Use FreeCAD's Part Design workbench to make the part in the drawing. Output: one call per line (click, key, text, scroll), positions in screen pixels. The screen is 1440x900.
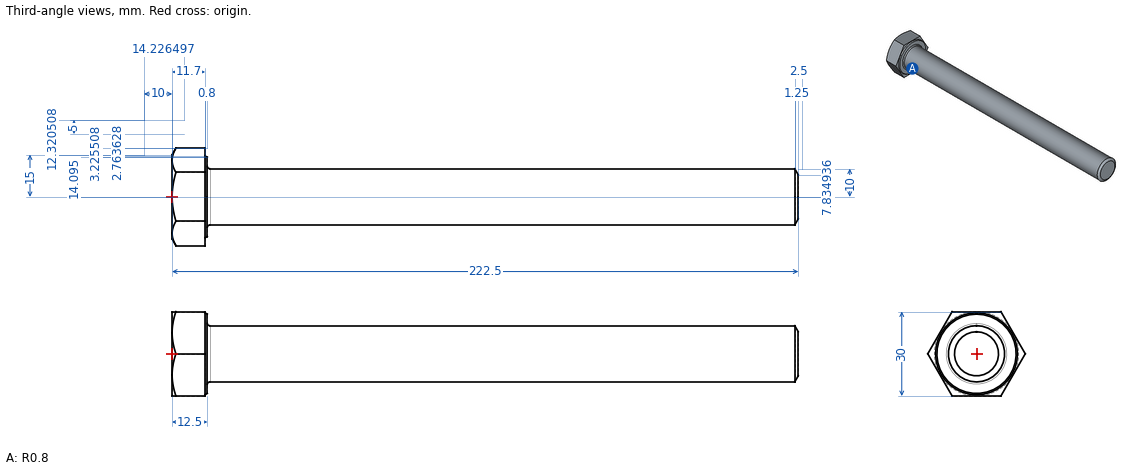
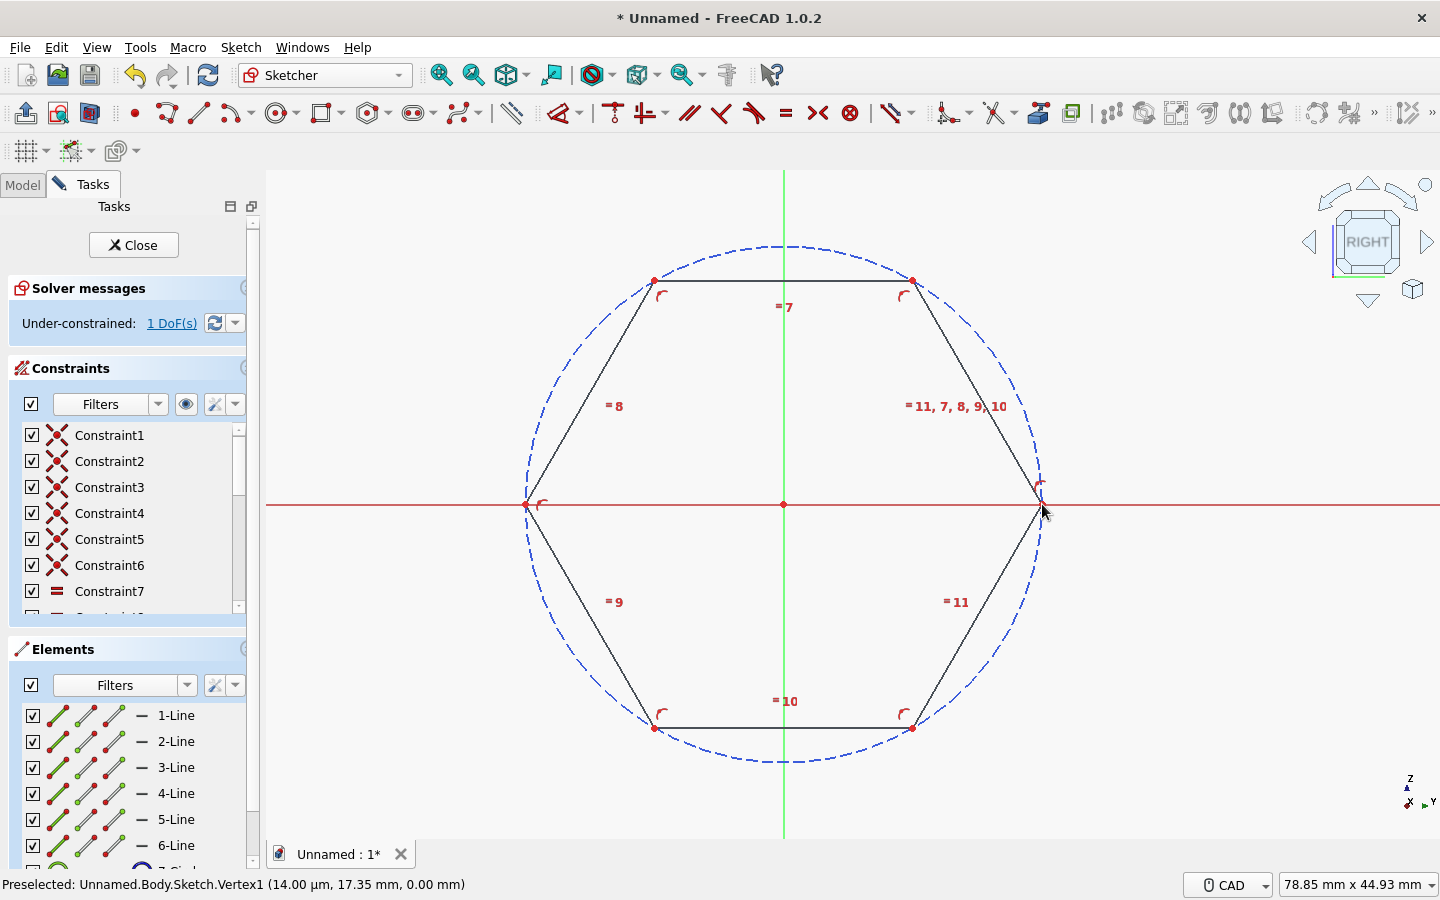
click(558, 114)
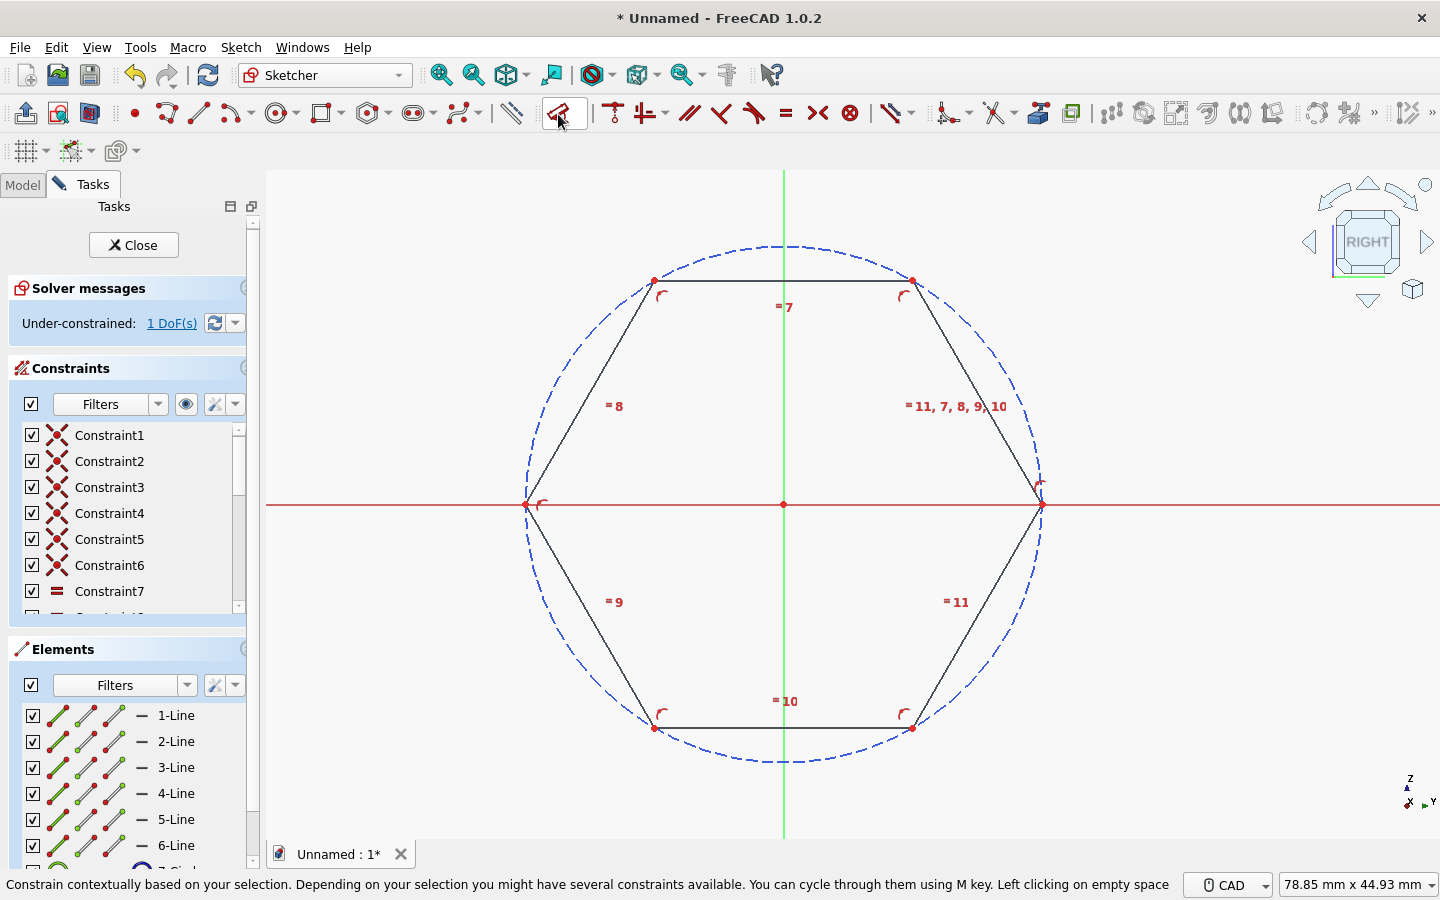
click(655, 728)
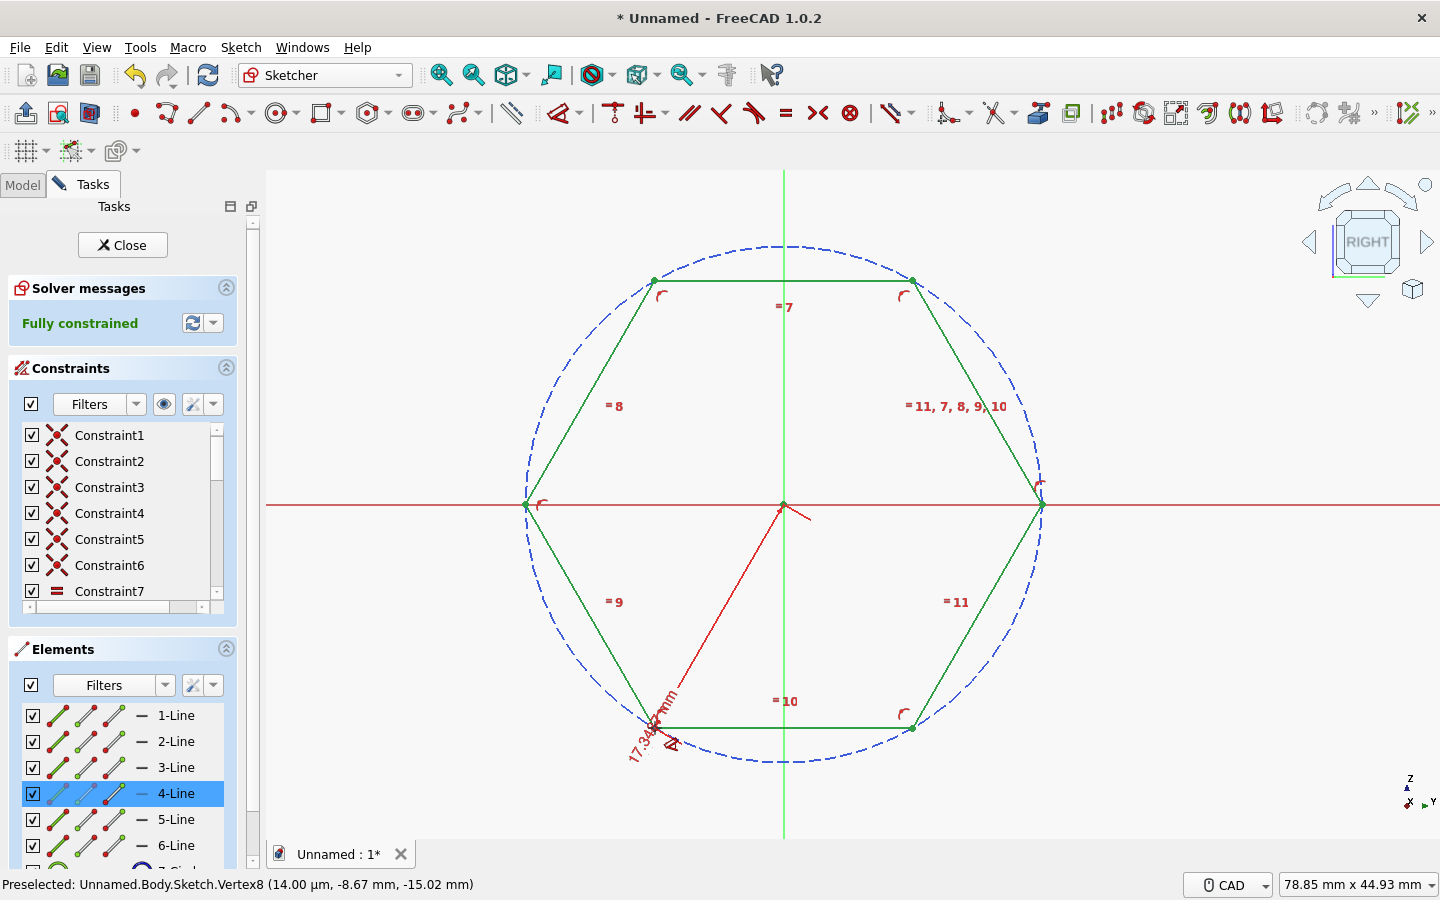
click(913, 281)
click(947, 402)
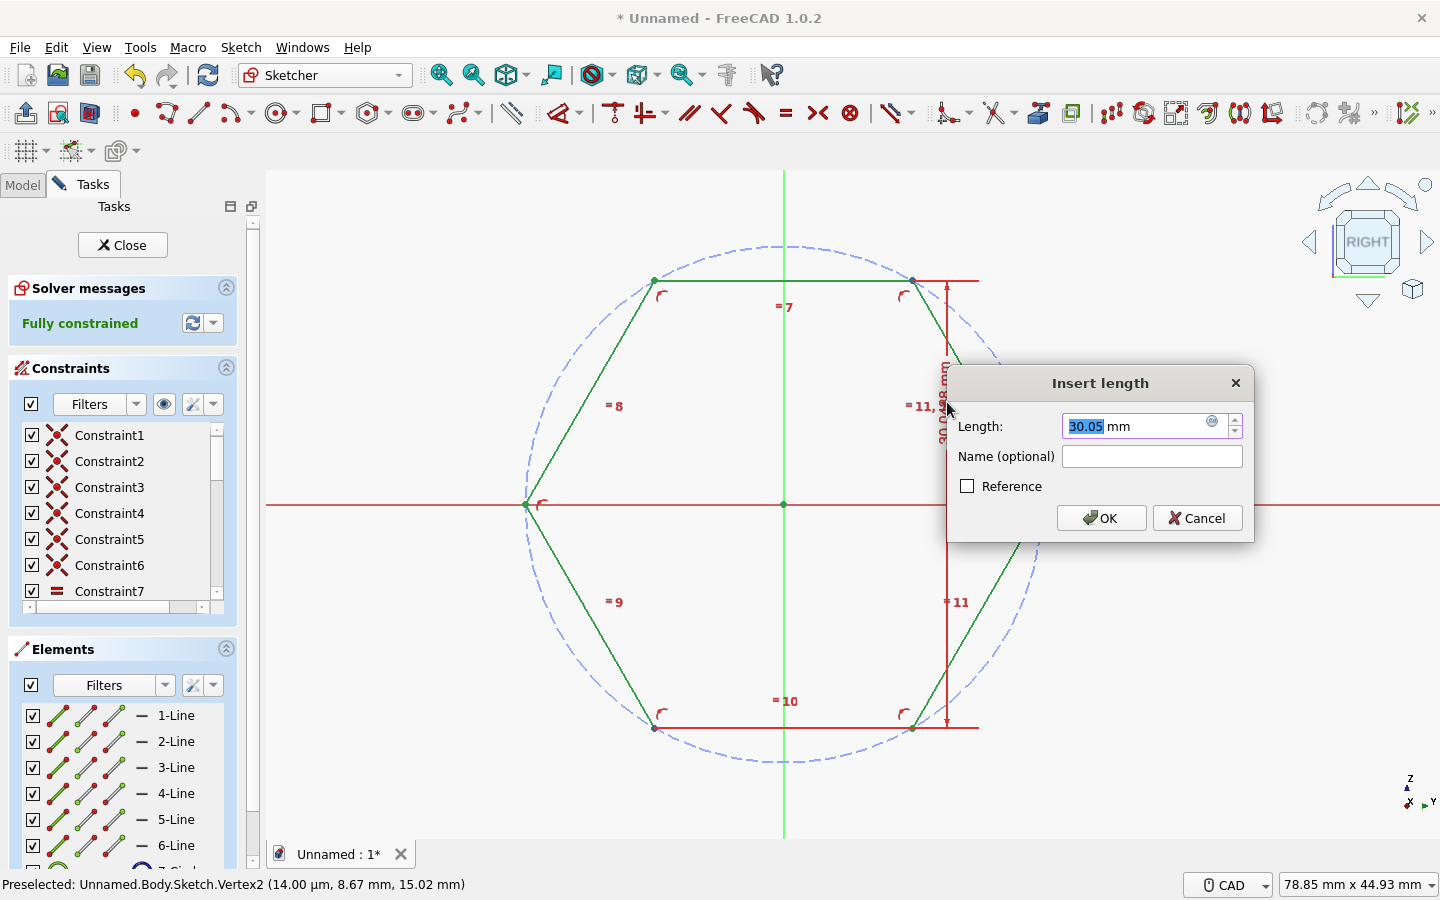
text(30)
key(Return)
key(Escape)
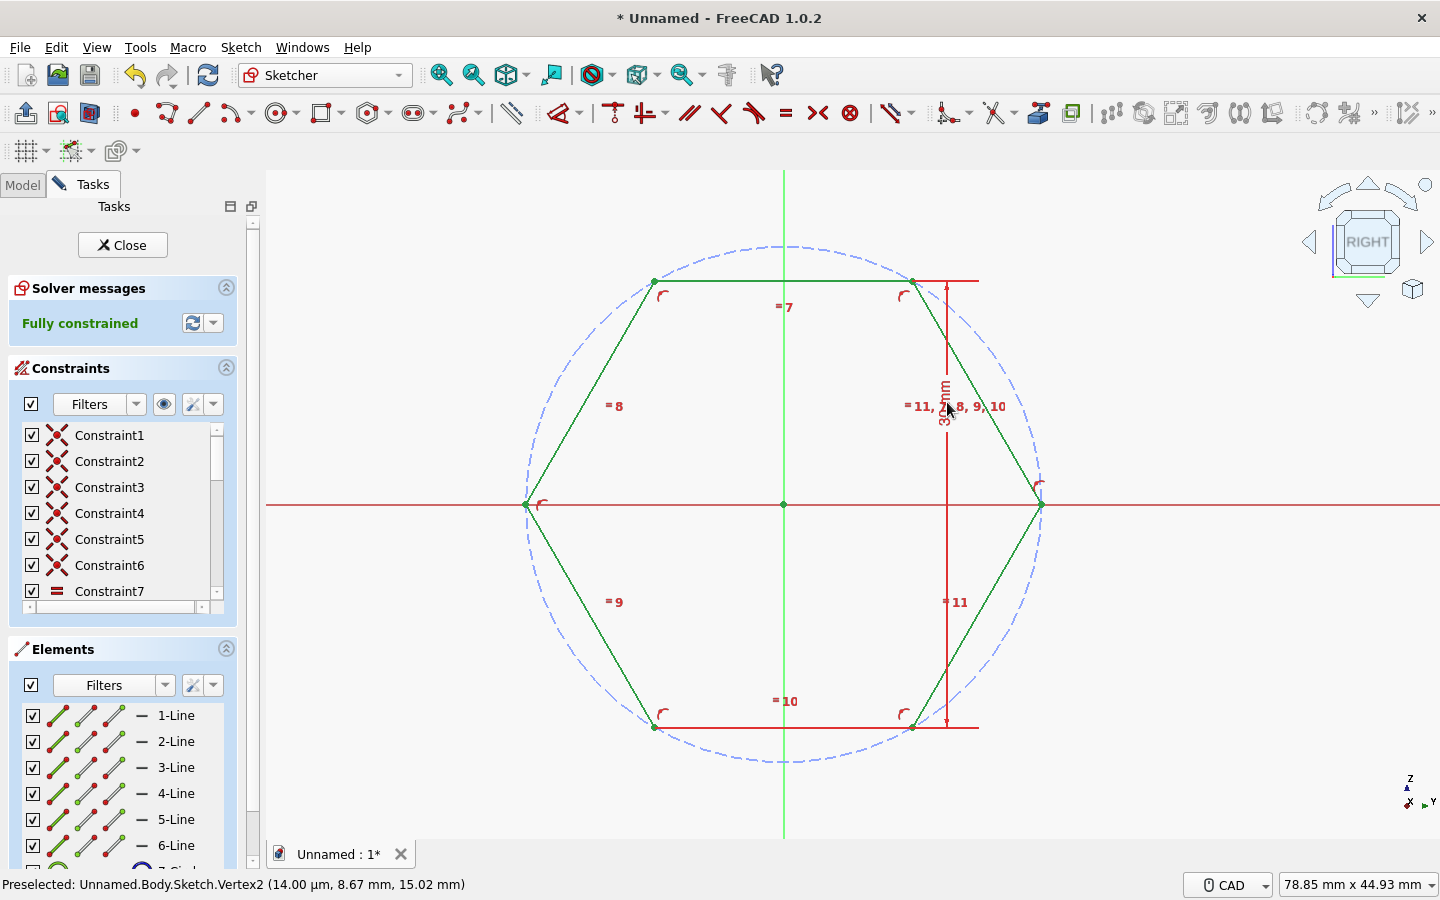
click(123, 245)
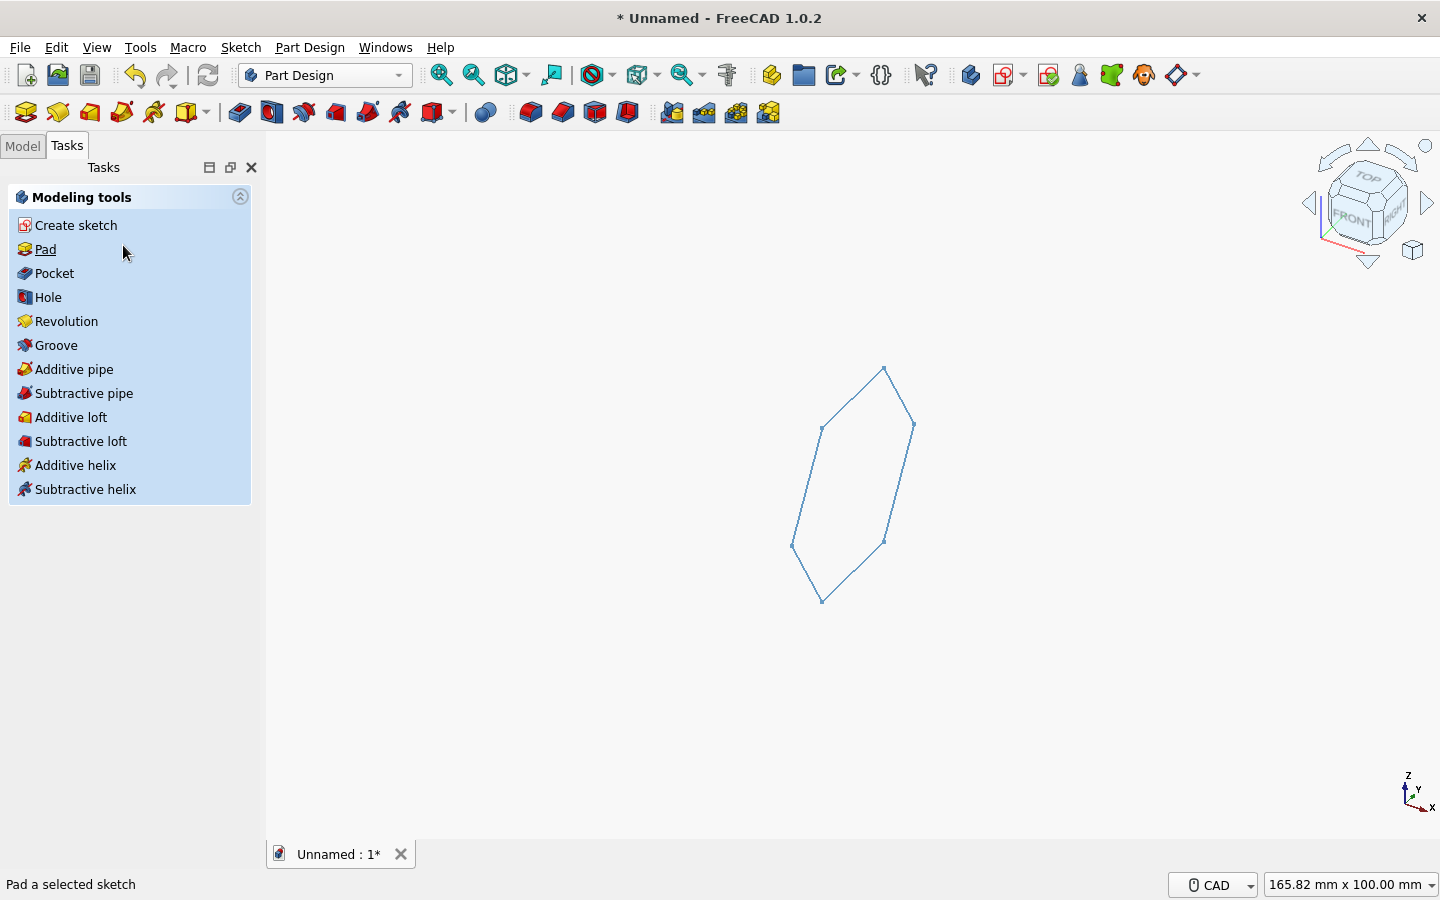
click(26, 112)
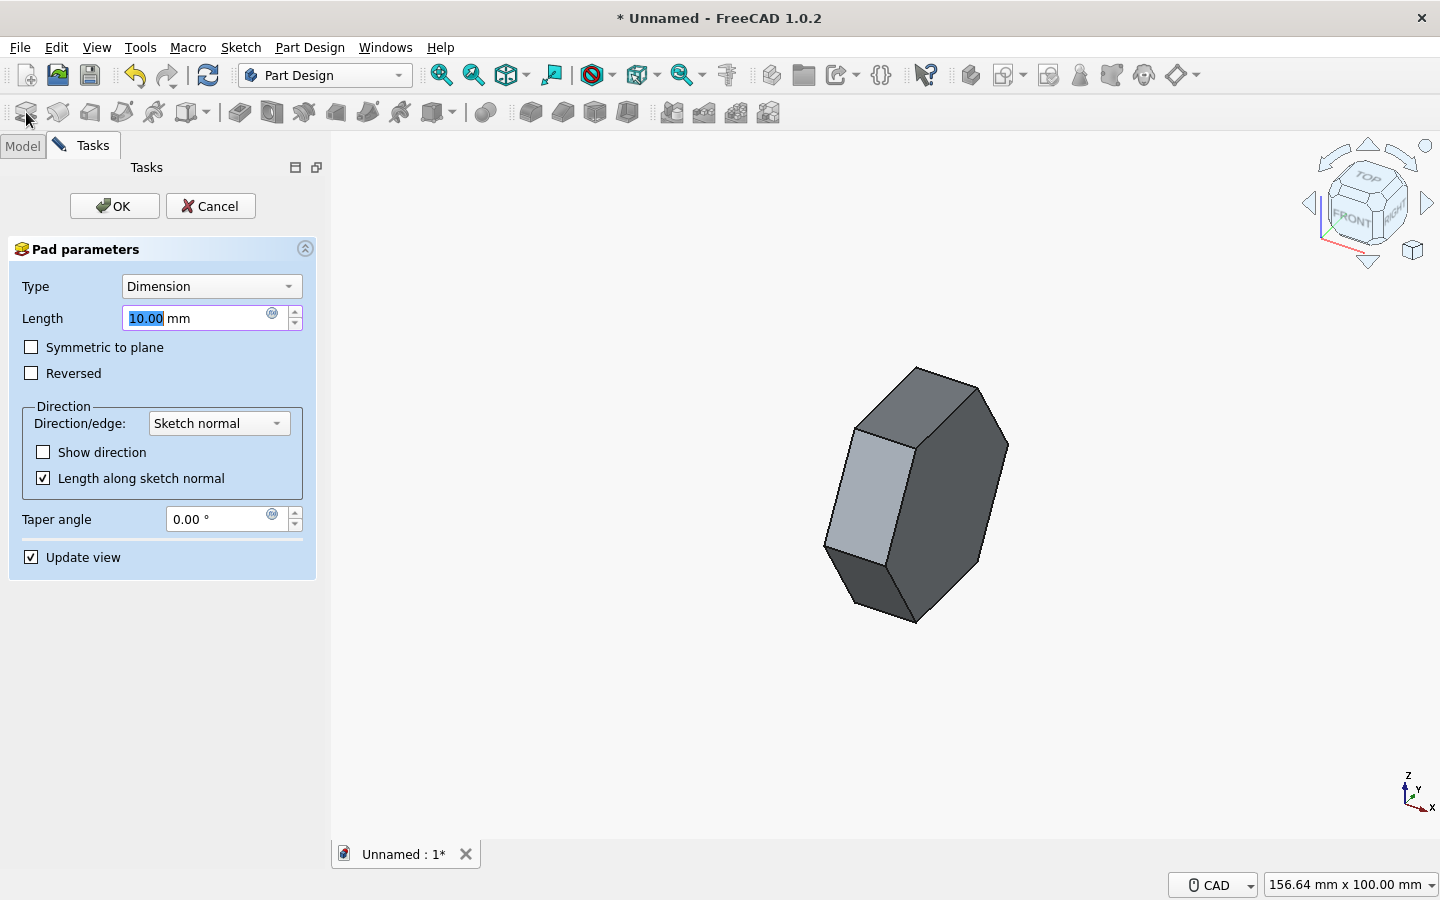
text(12.5)
key(Tab)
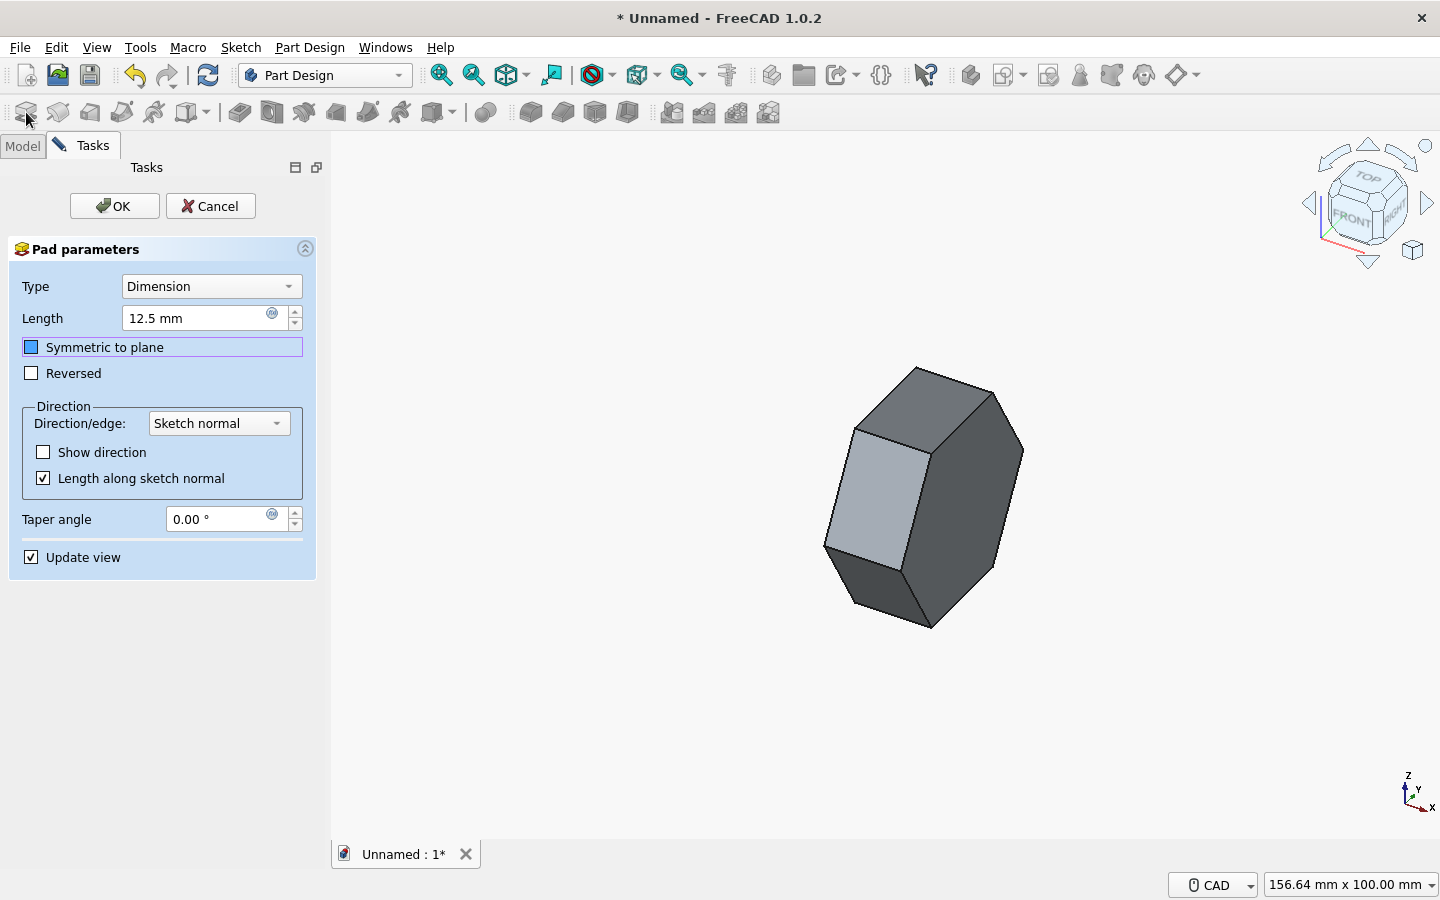
click(115, 206)